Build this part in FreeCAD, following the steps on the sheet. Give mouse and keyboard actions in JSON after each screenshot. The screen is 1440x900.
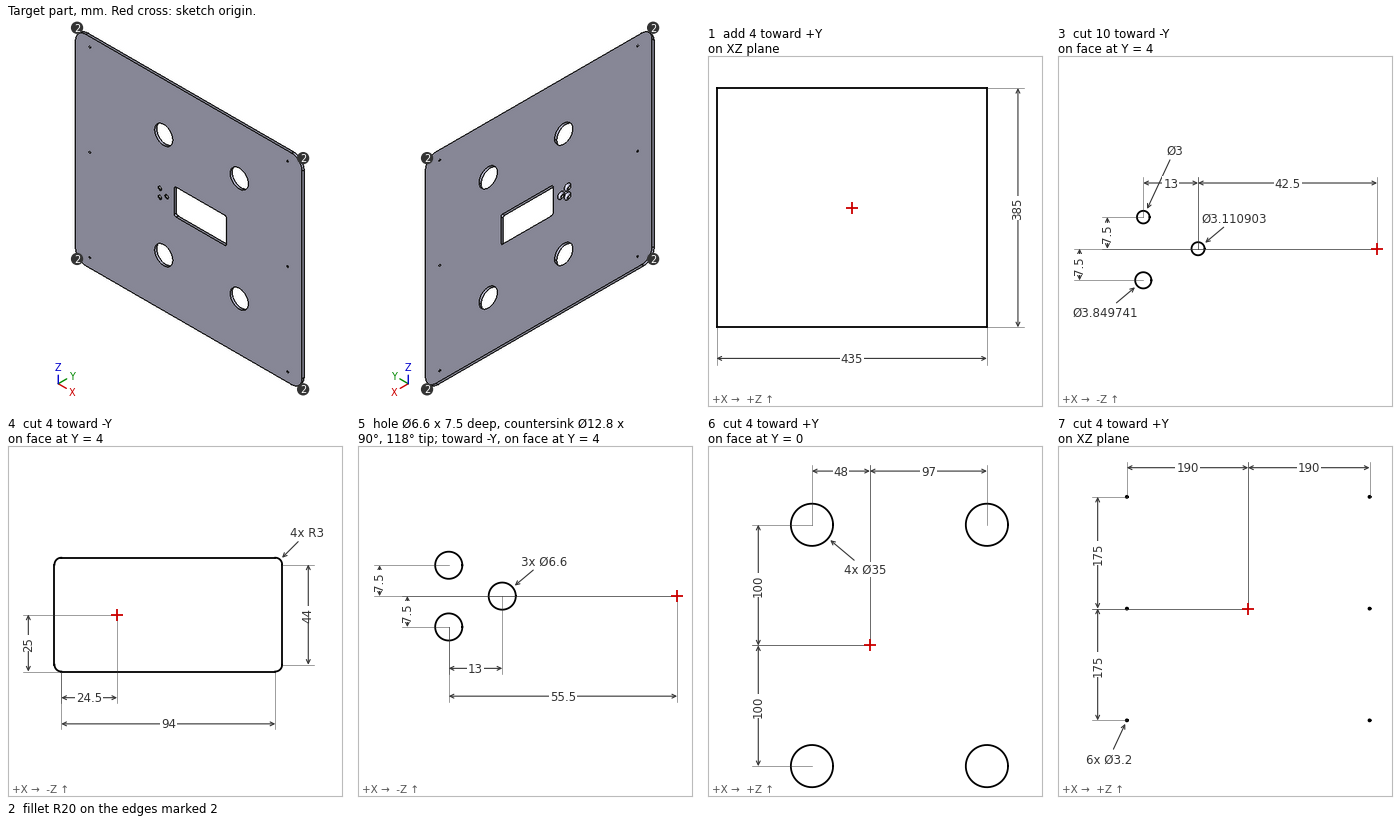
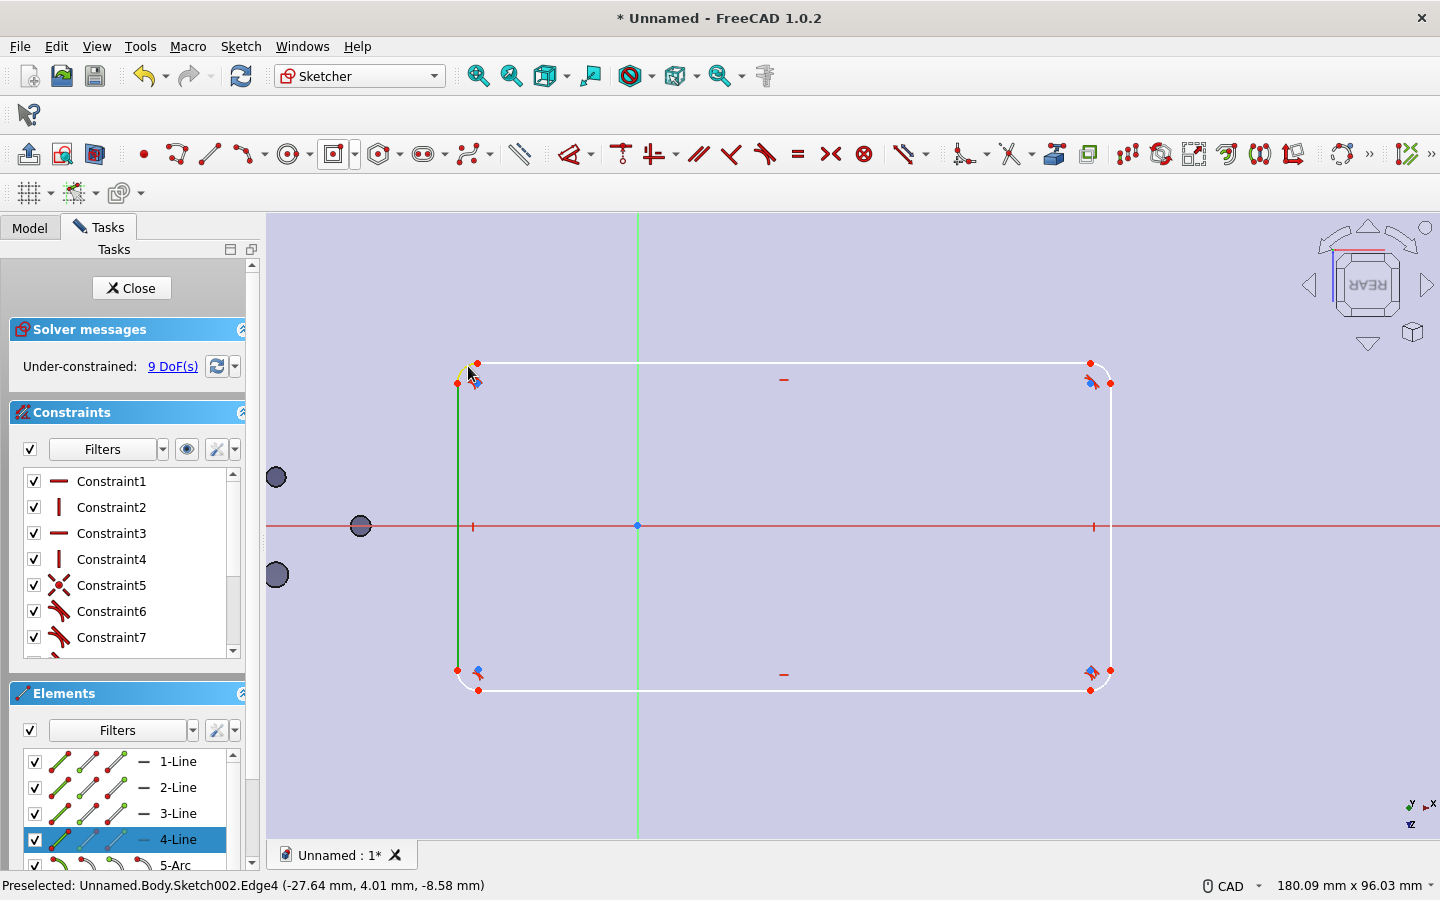
{"action": "scroll", "coordinate": [460, 680], "scroll_direction": "up", "scroll_amount": 2}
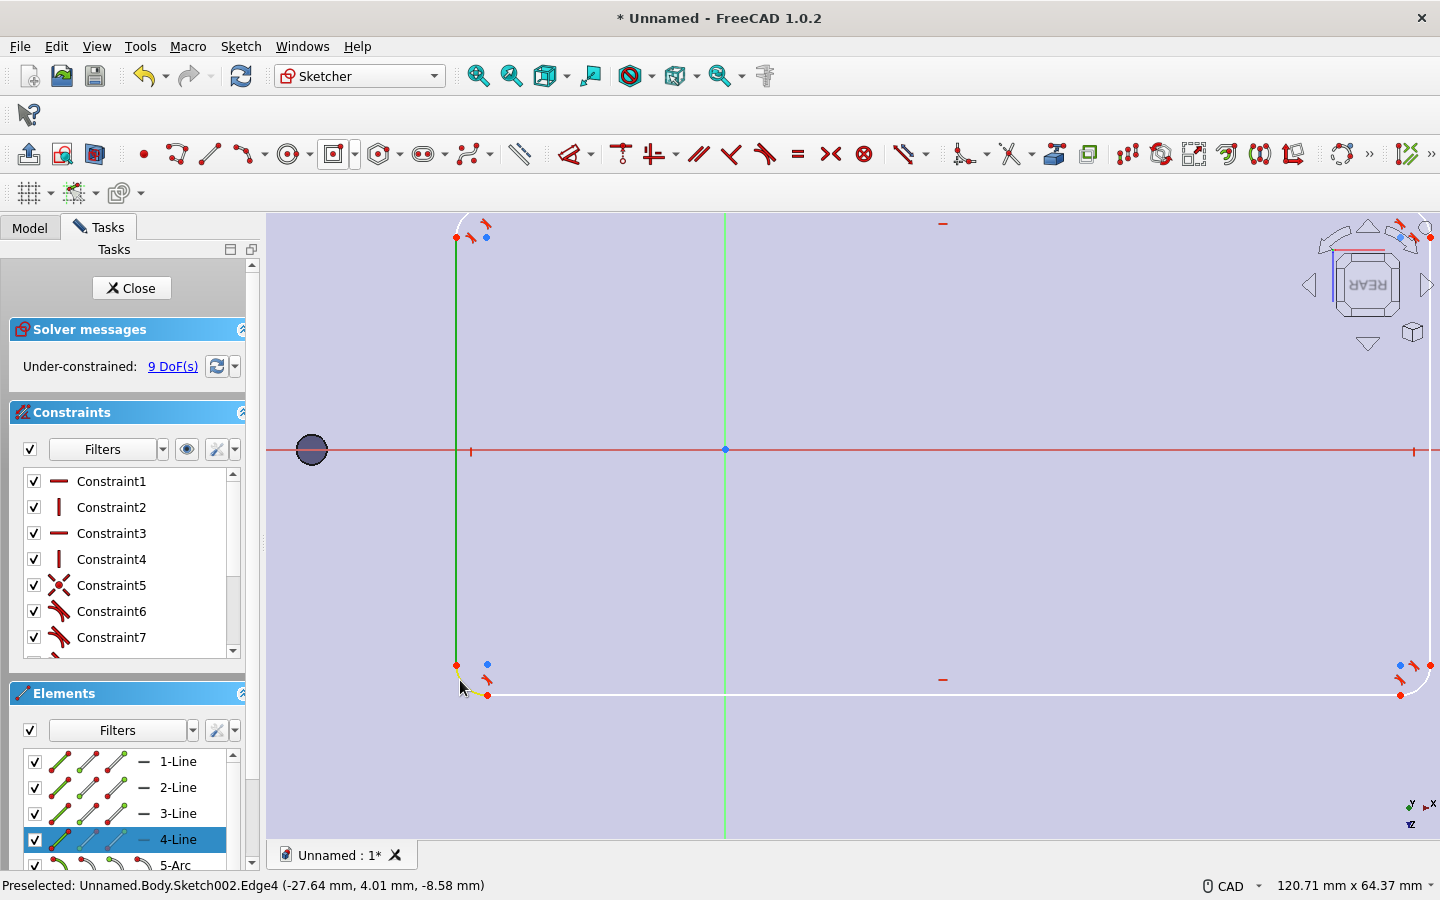
{"action": "left_click", "coordinate": [460, 679]}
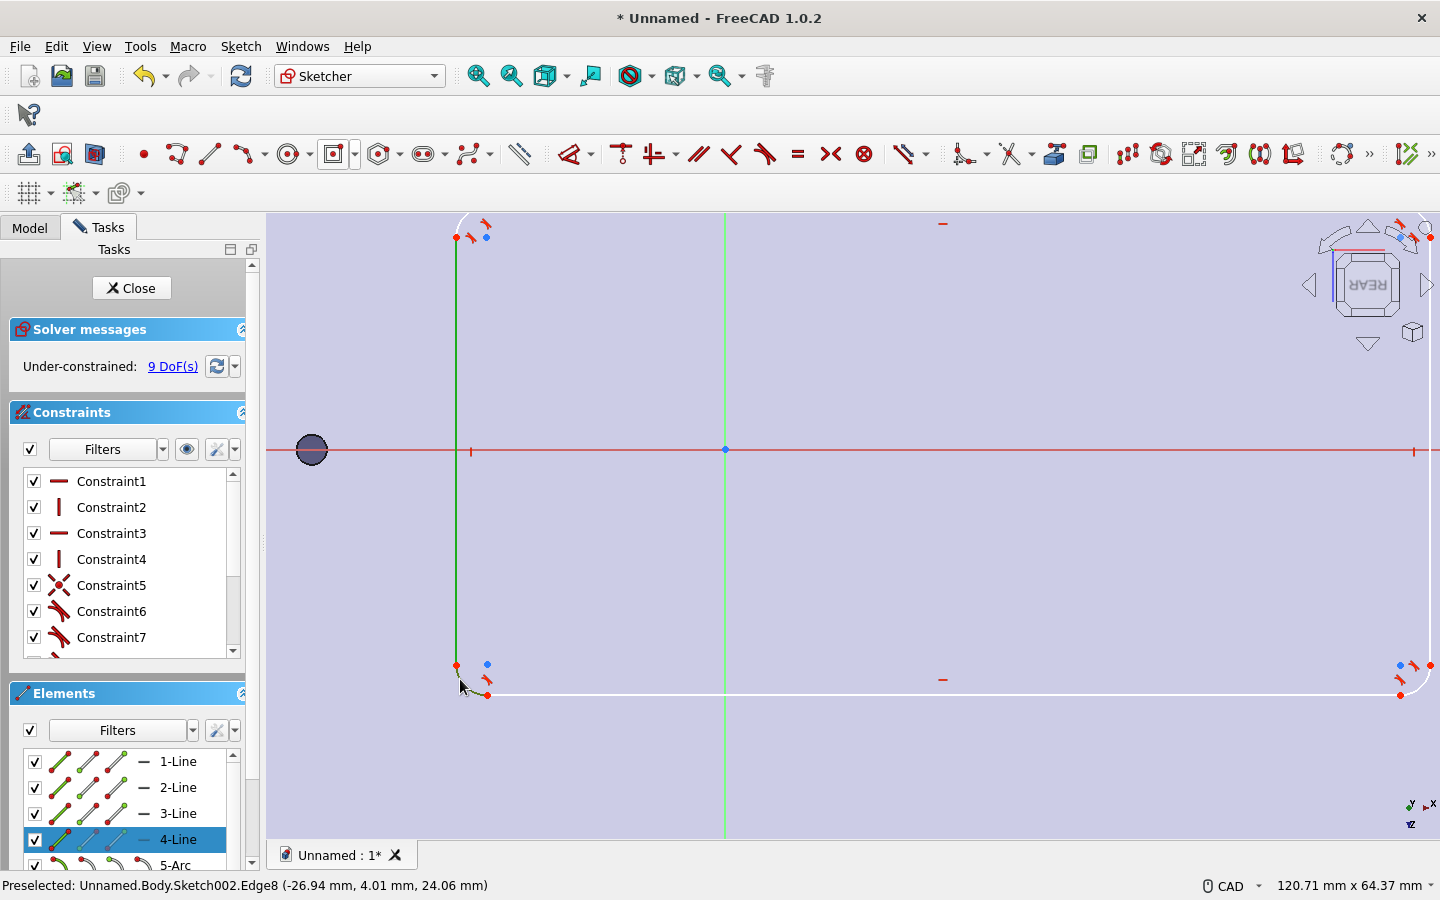
{"action": "left_click", "coordinate": [765, 154]}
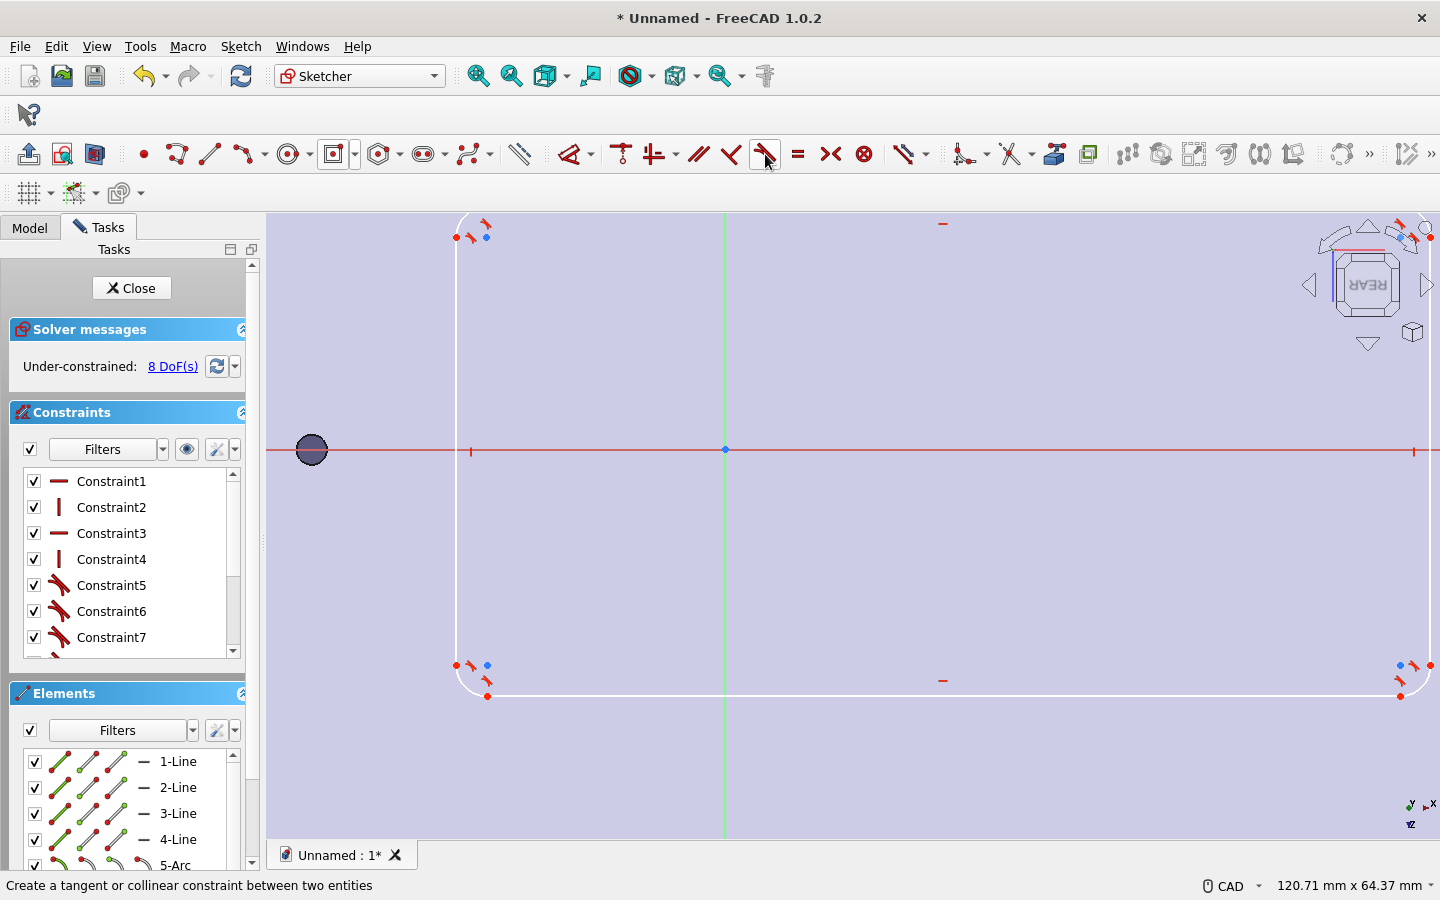
{"action": "scroll", "coordinate": [460, 681], "scroll_direction": "down", "scroll_amount": 2}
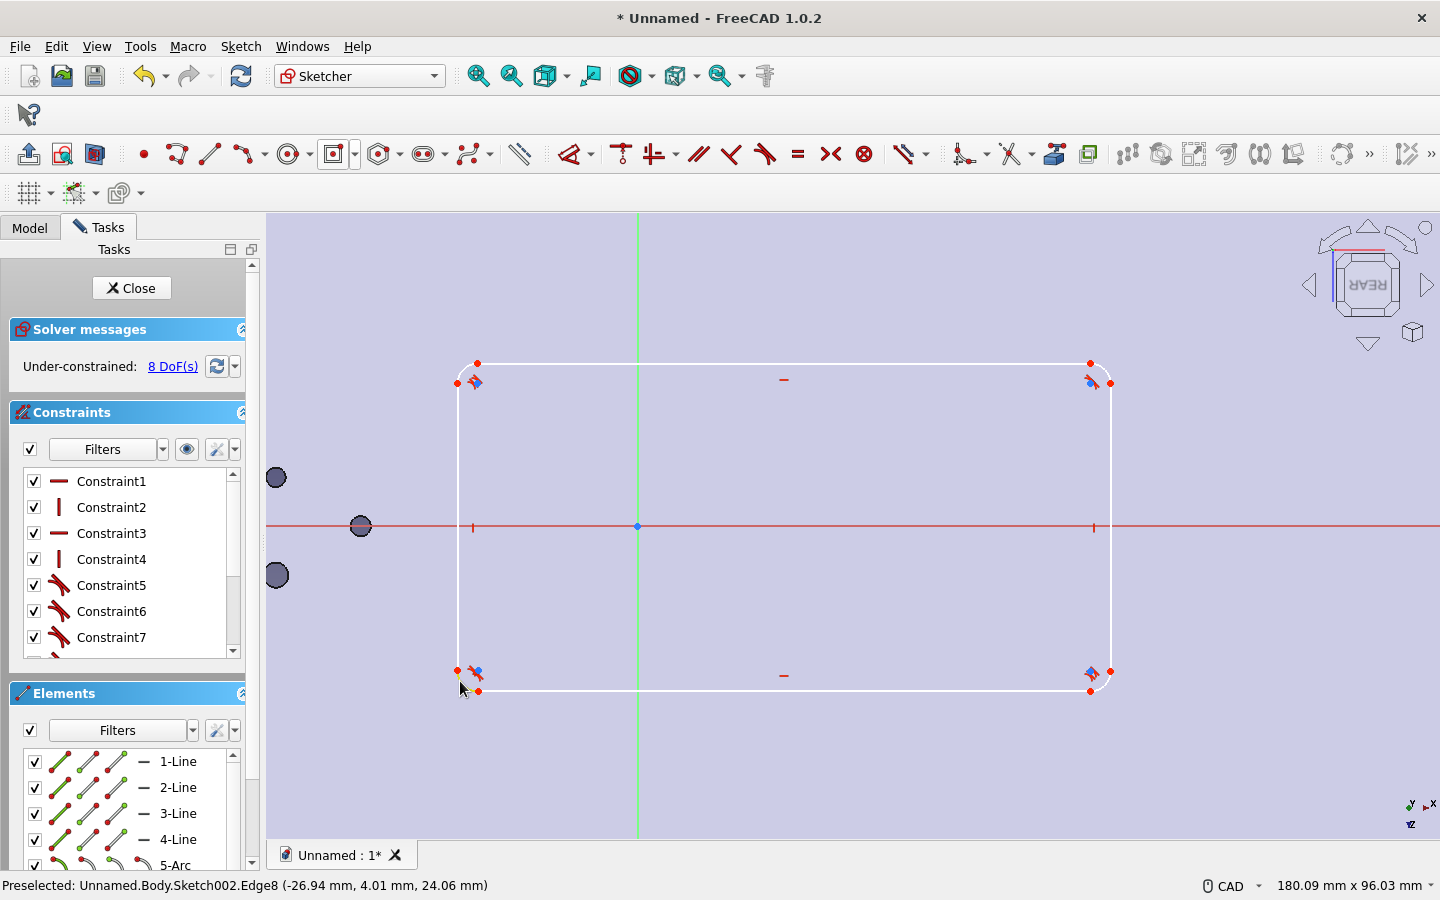
{"action": "scroll", "coordinate": [1099, 689], "scroll_direction": "up", "scroll_amount": 2}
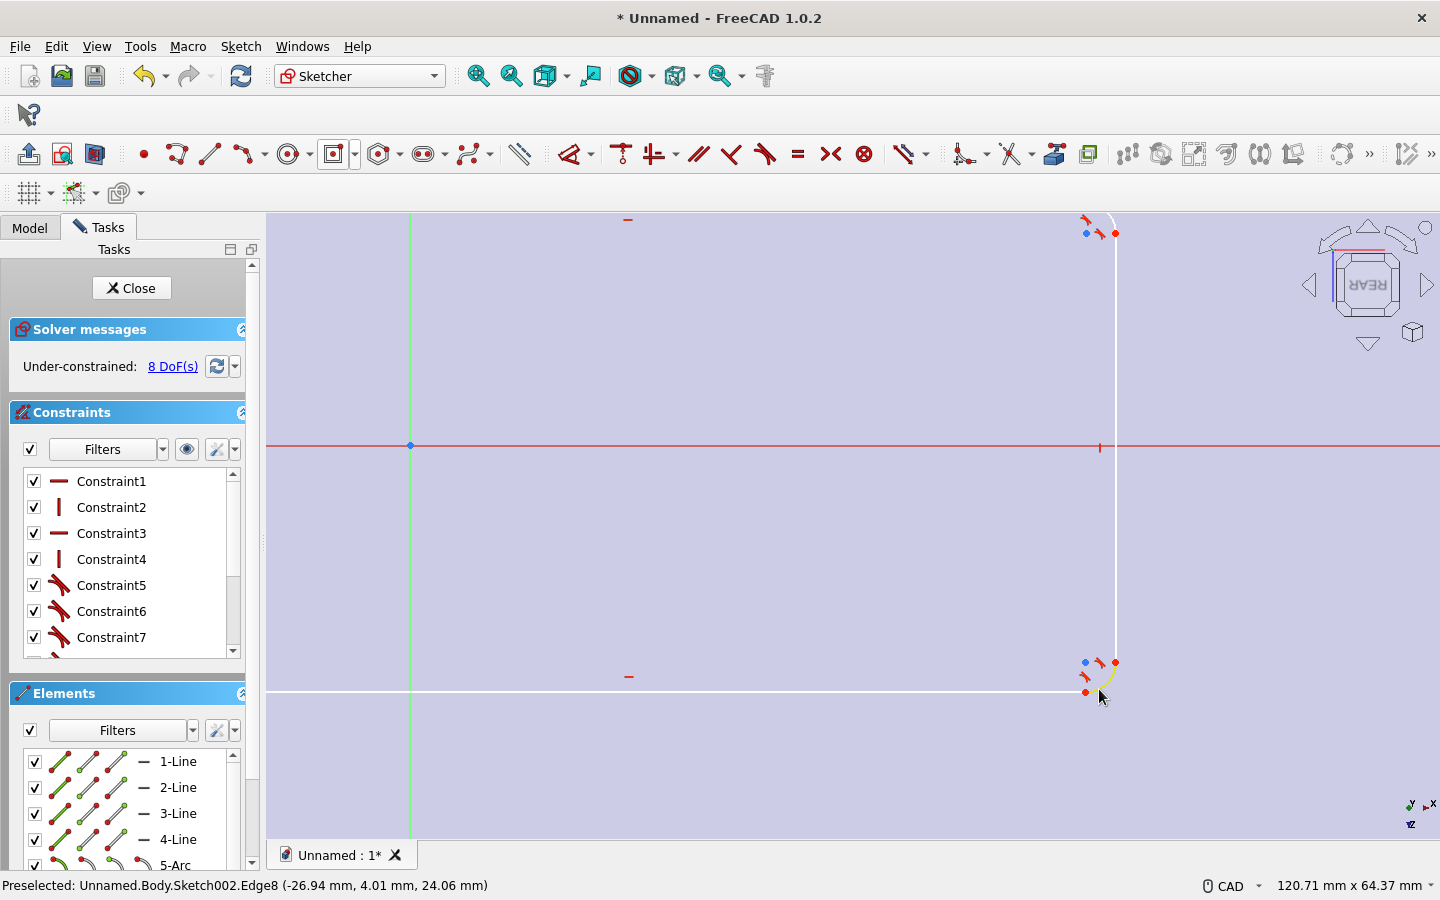
{"action": "left_click", "coordinate": [1099, 689]}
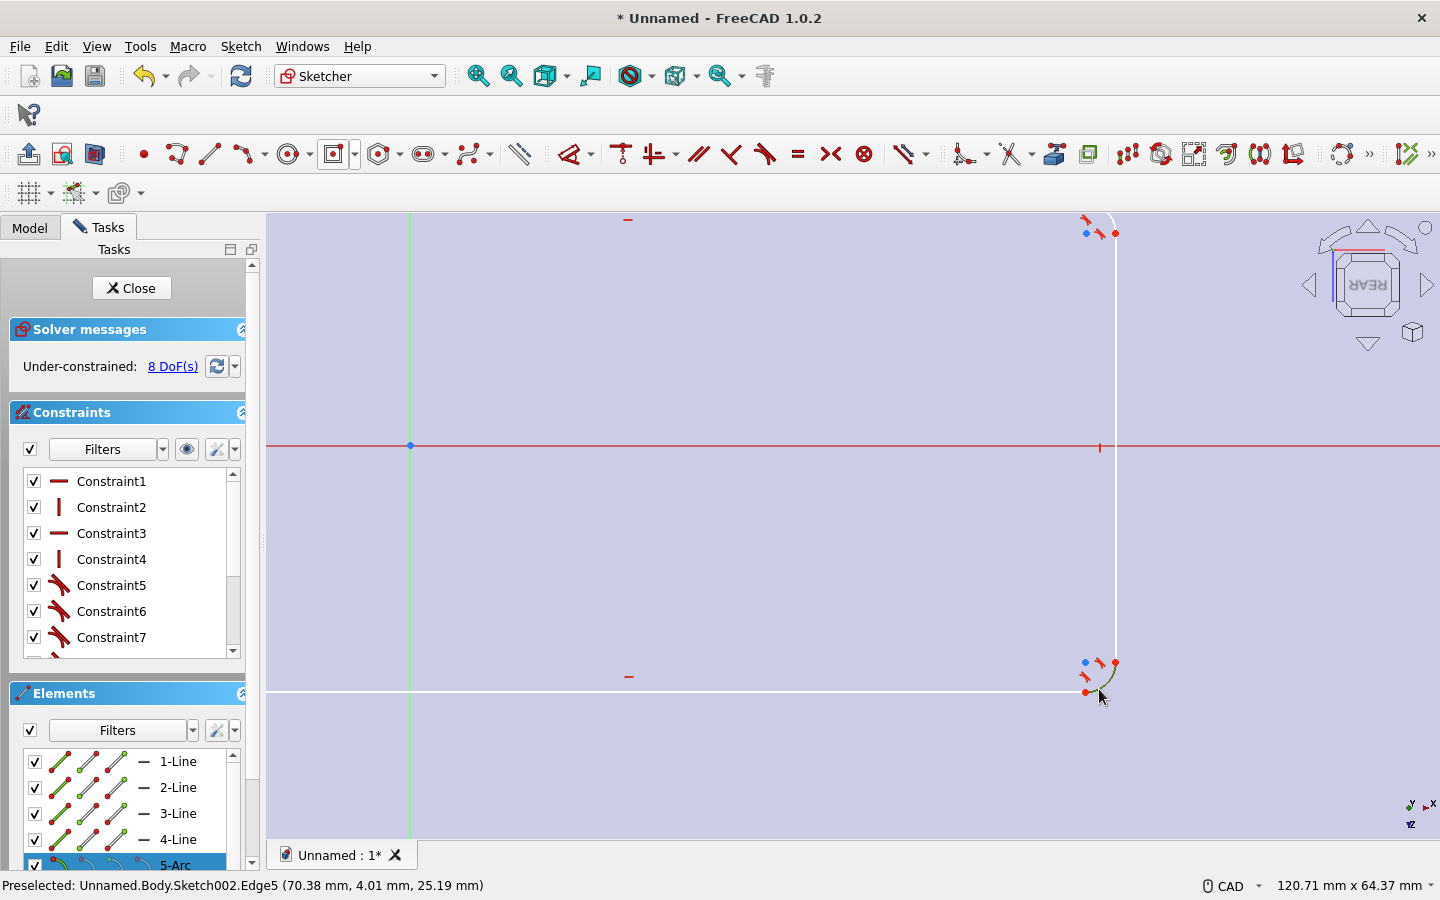
{"action": "scroll", "coordinate": [1100, 689], "scroll_direction": "down", "scroll_amount": 2}